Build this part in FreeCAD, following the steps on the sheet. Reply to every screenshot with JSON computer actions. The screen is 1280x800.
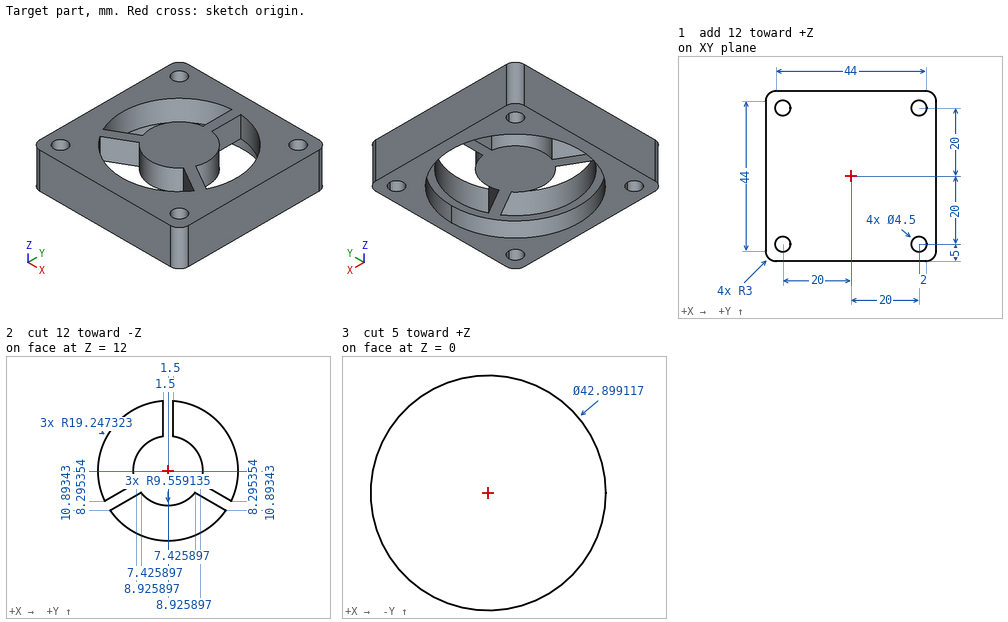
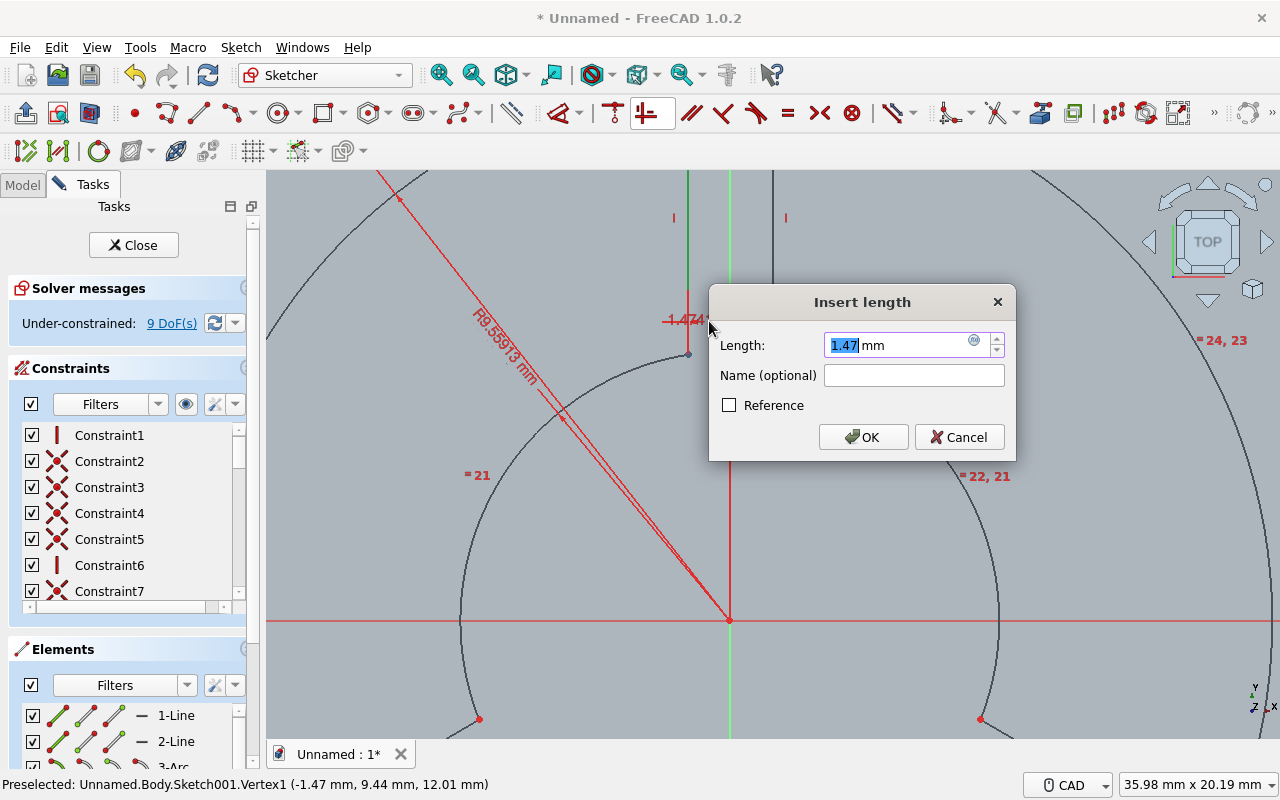
{"action": "type", "text": "1.5"}
{"action": "key", "text": "Return"}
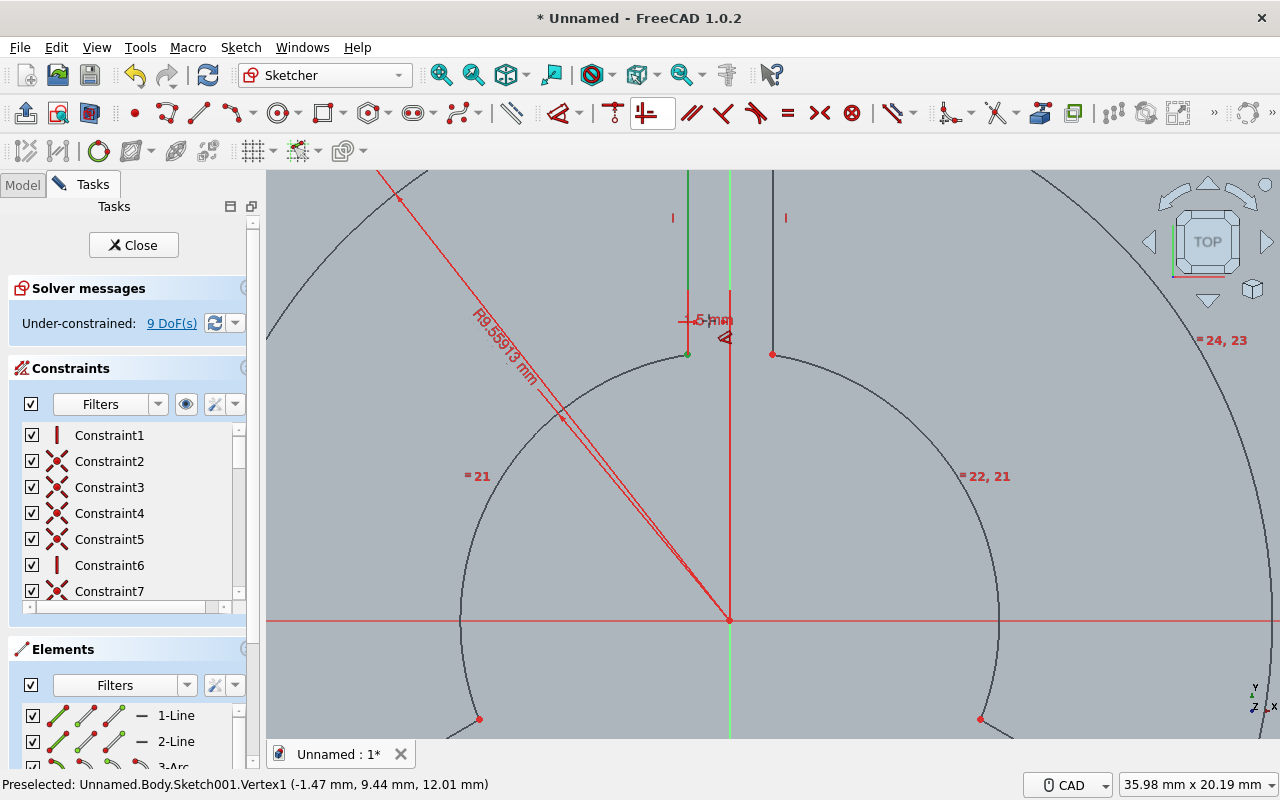
{"action": "scroll", "coordinate": [690, 357], "scroll_direction": "down", "scroll_amount": 5}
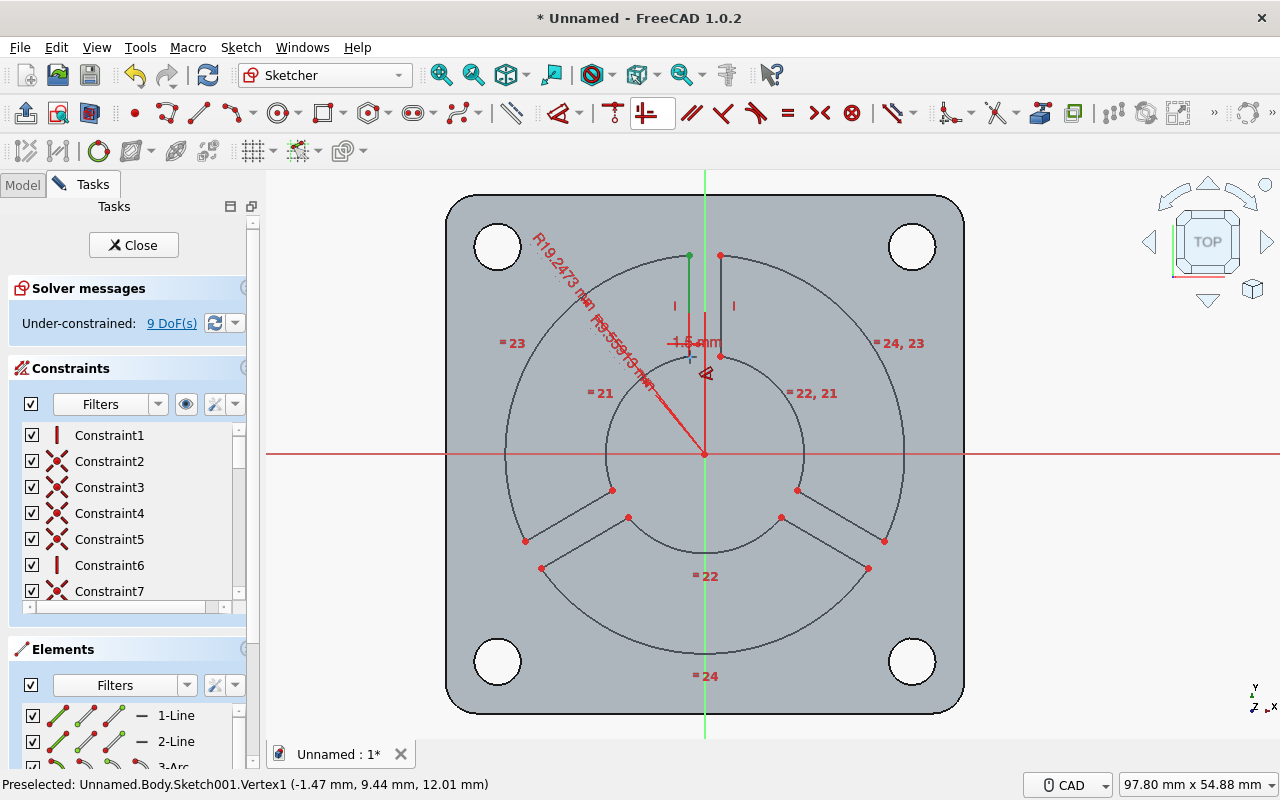
{"action": "scroll", "coordinate": [721, 255], "scroll_direction": "up", "scroll_amount": 5}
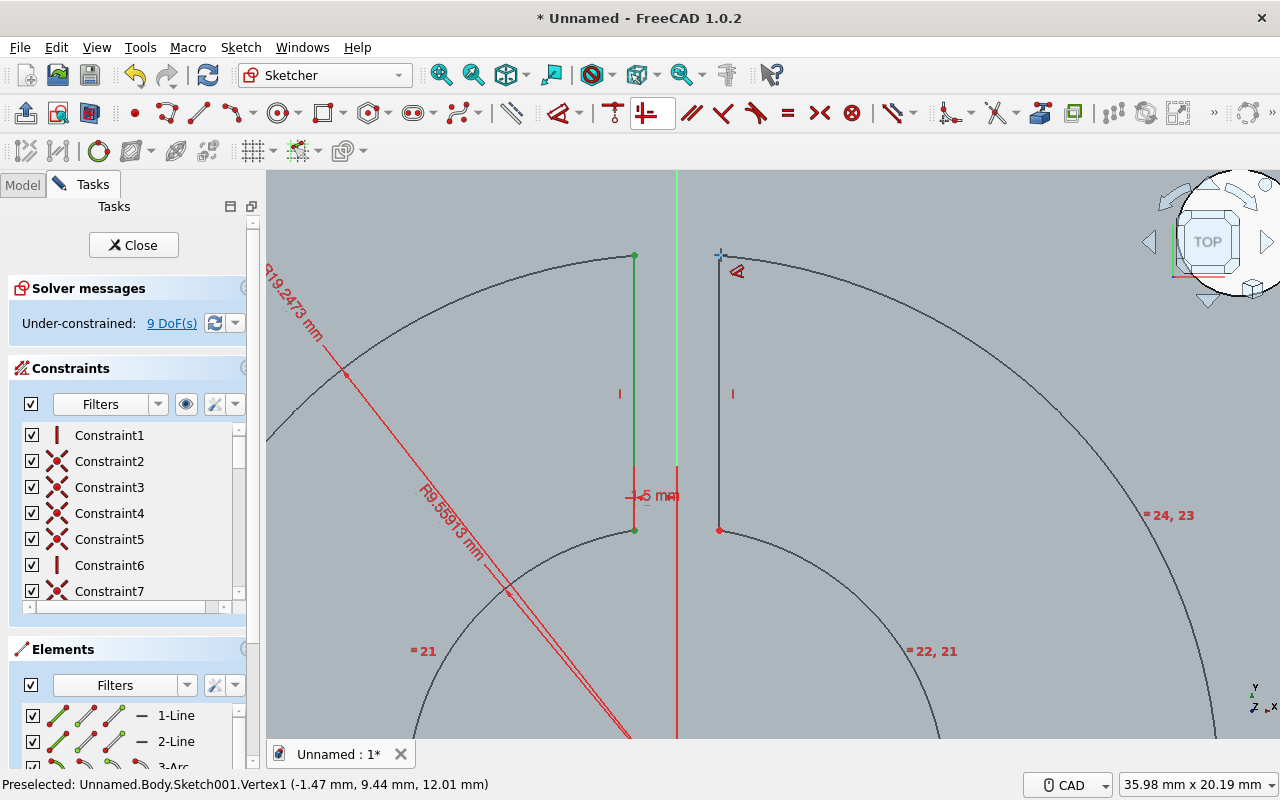
{"action": "left_click", "coordinate": [719, 256]}
{"action": "left_click", "coordinate": [698, 222]}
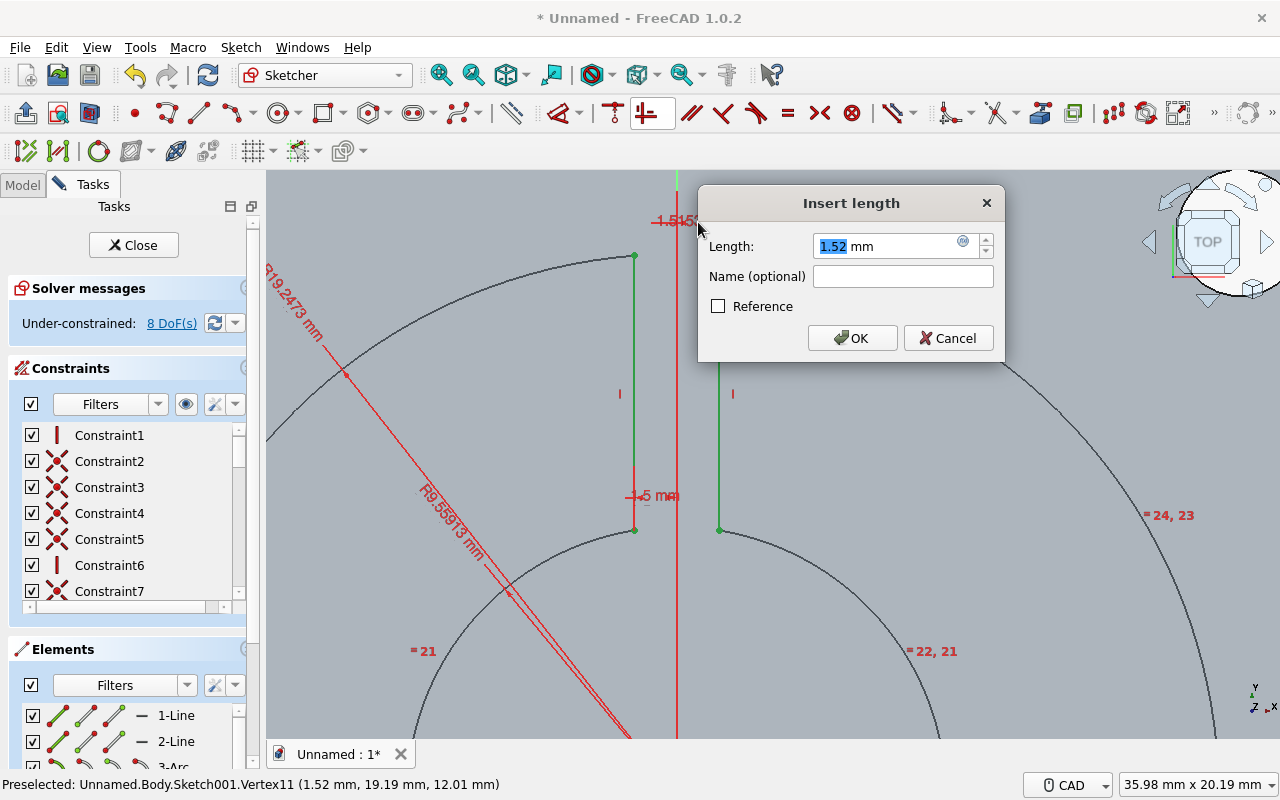
{"action": "type", "text": "1.5"}
{"action": "key", "text": "Return"}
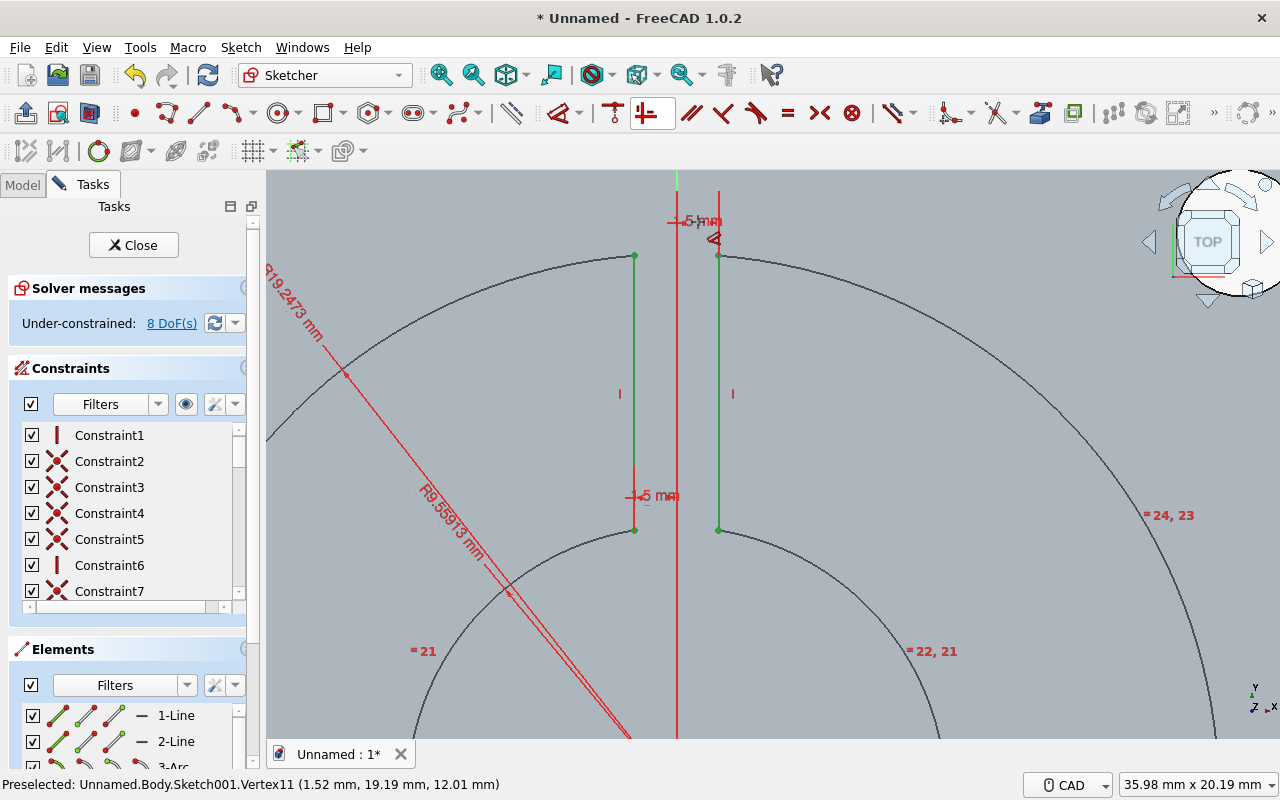
{"action": "scroll", "coordinate": [721, 255], "scroll_direction": "down", "scroll_amount": 5}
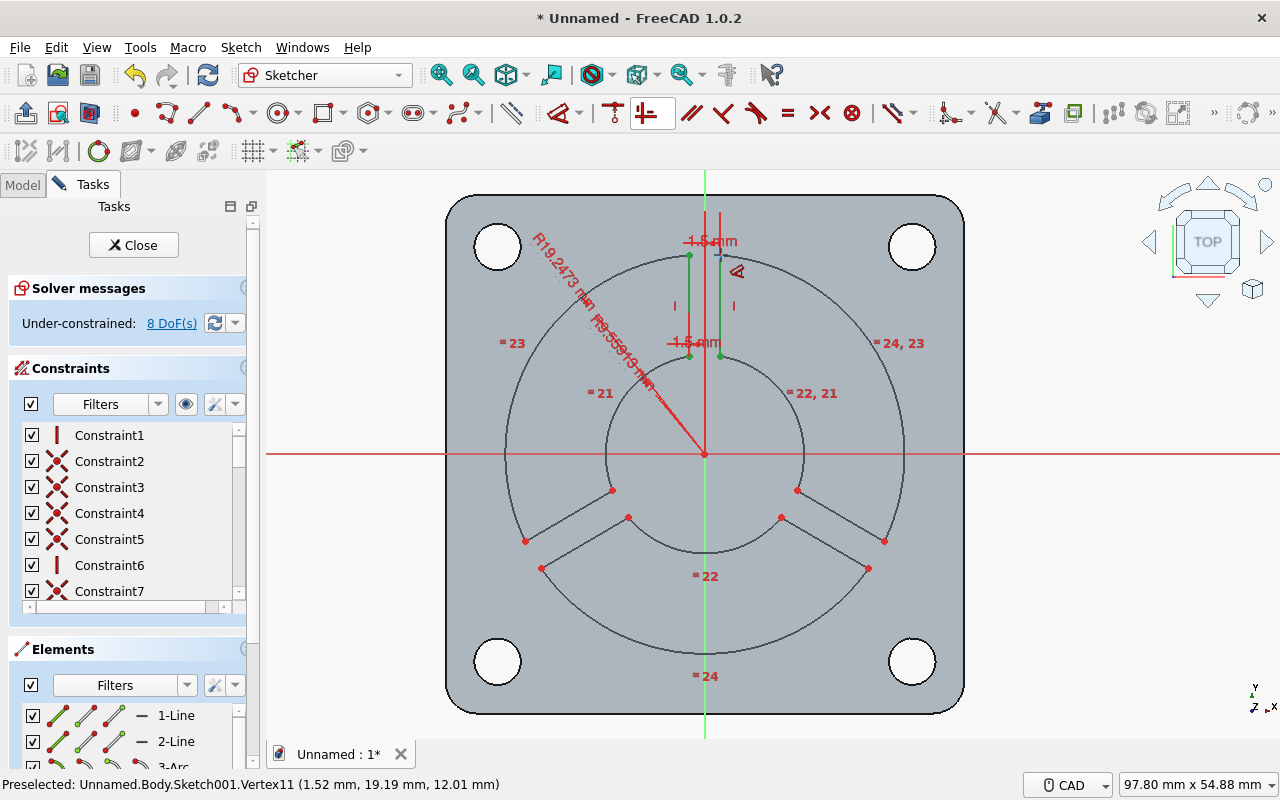
{"action": "left_click", "coordinate": [525, 542]}
{"action": "left_click", "coordinate": [491, 498]}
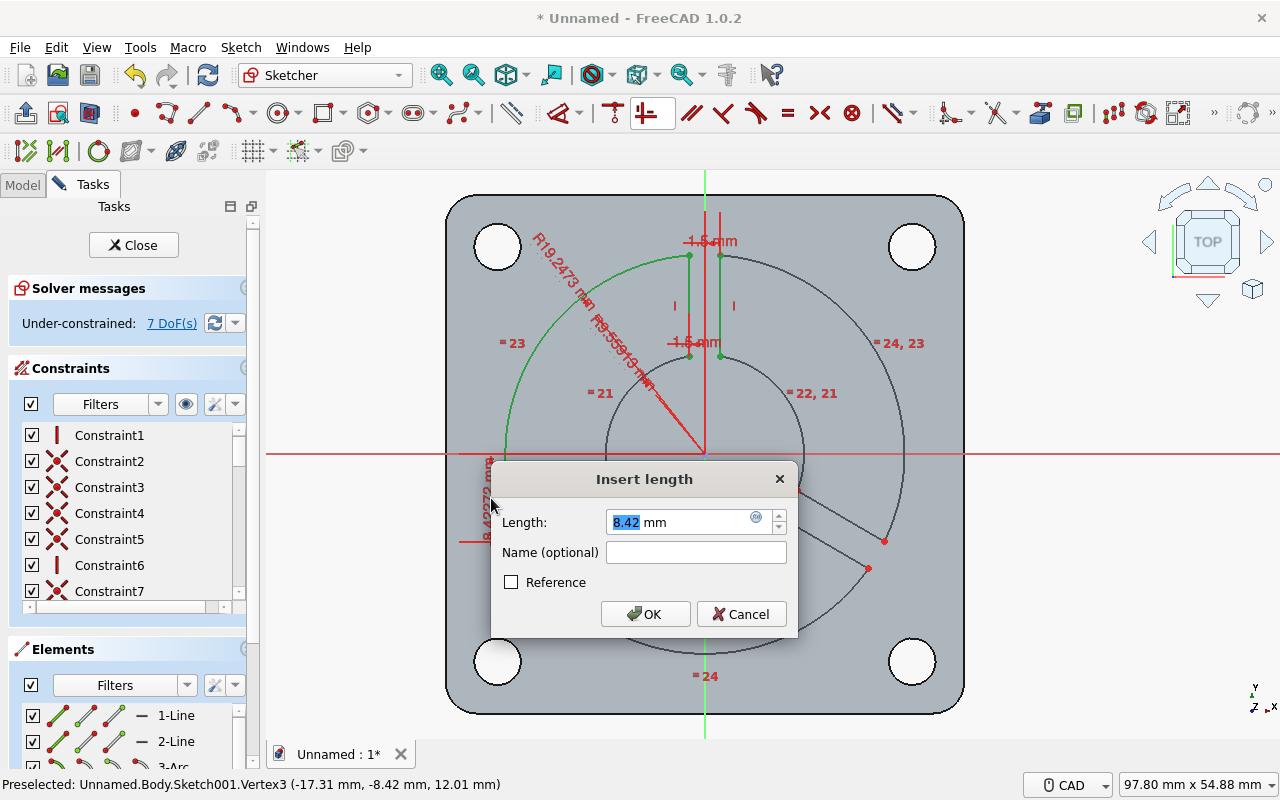
{"action": "type", "text": "8.295354"}
{"action": "key", "text": "Return"}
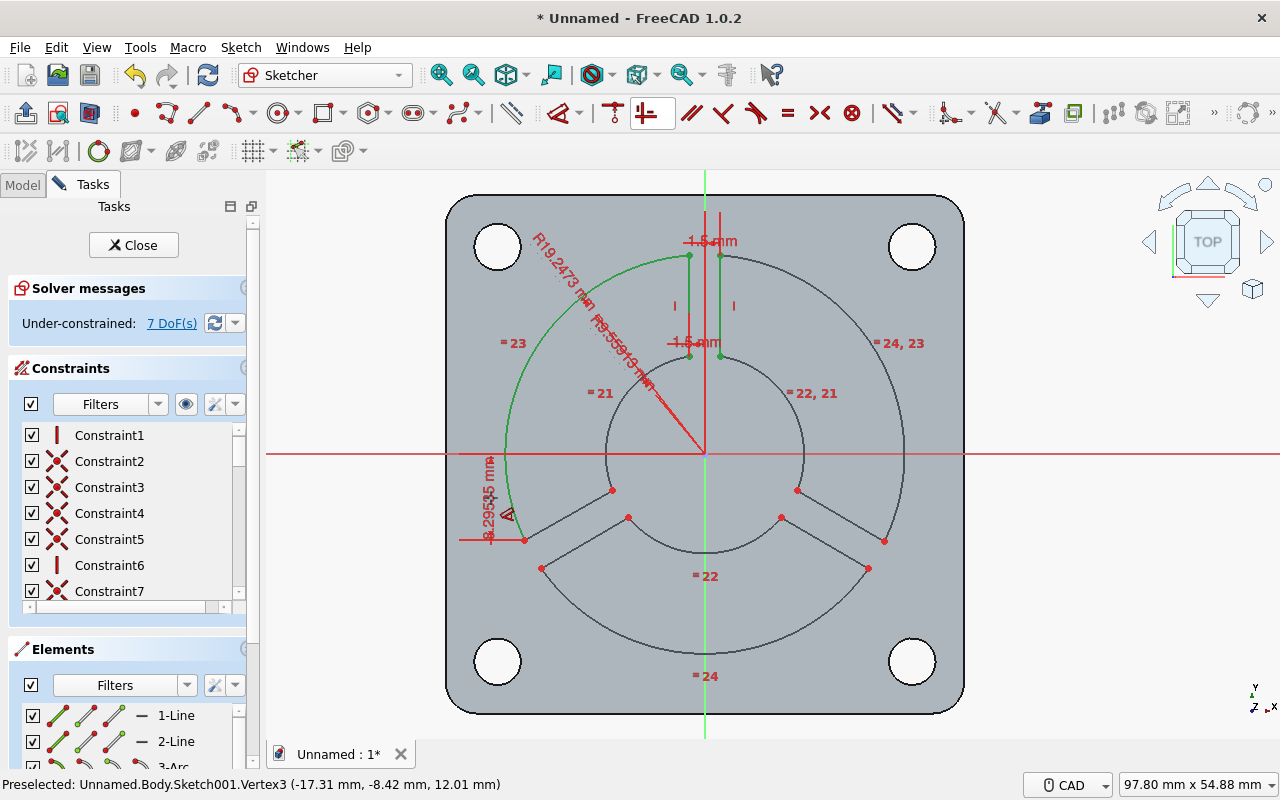
{"action": "left_click", "coordinate": [613, 491]}
{"action": "left_click", "coordinate": [659, 525]}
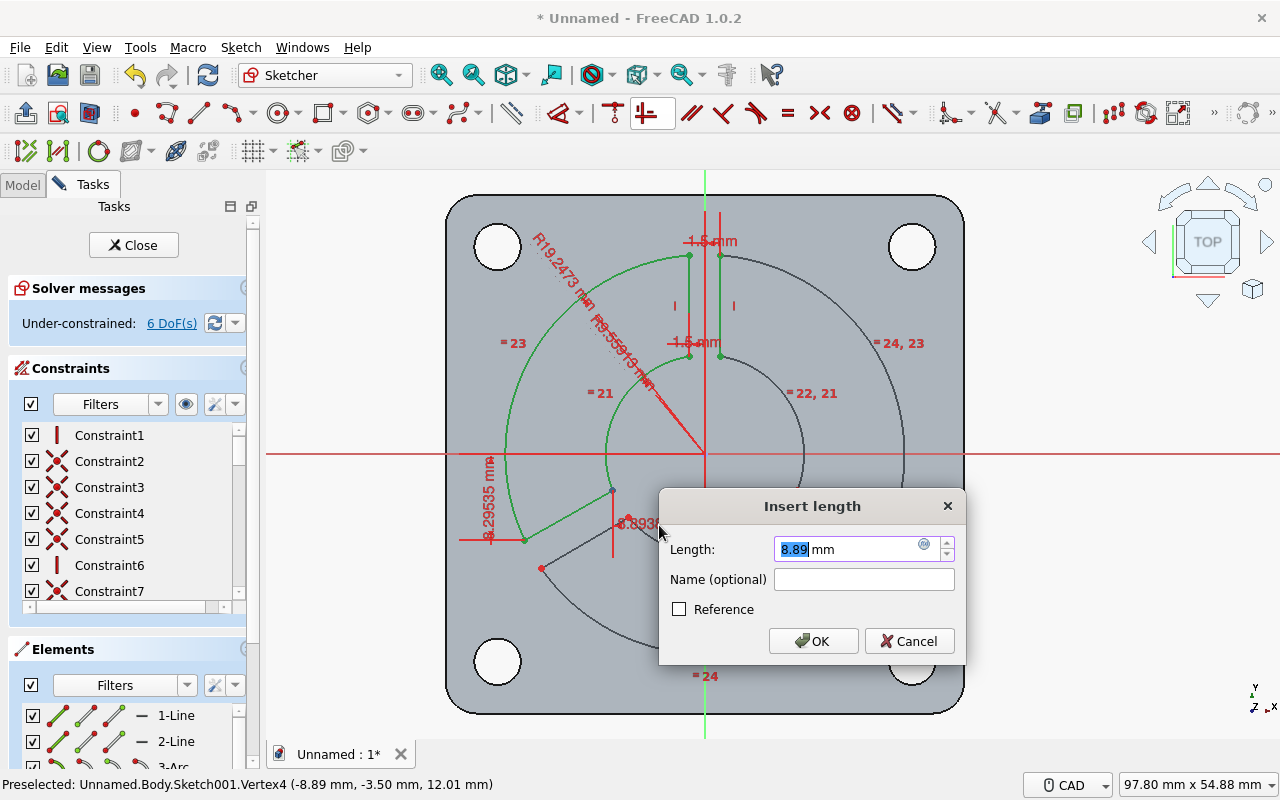
{"action": "type", "text": "8.925897"}
{"action": "key", "text": "Return"}